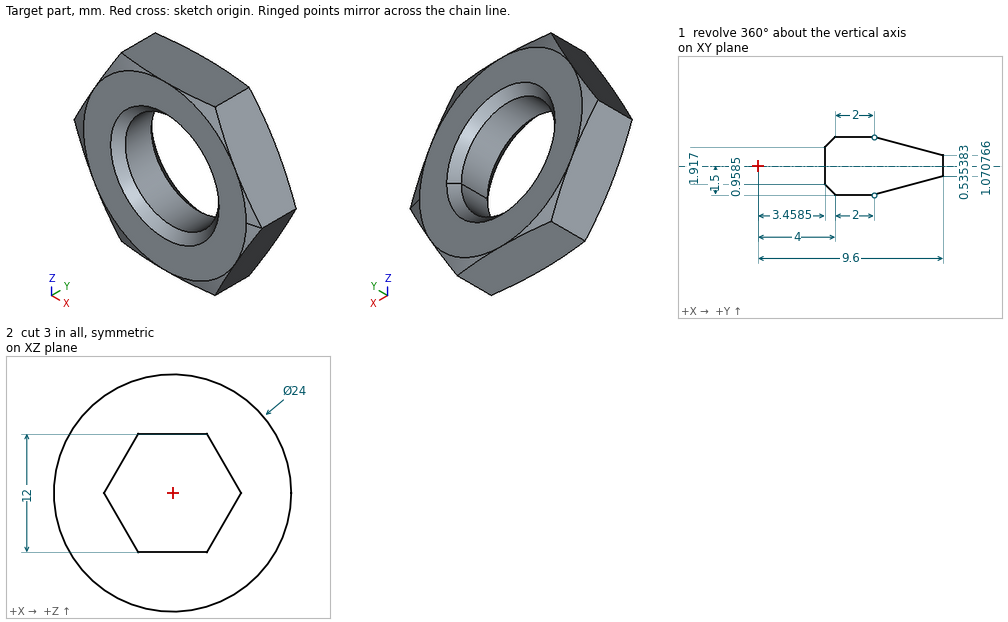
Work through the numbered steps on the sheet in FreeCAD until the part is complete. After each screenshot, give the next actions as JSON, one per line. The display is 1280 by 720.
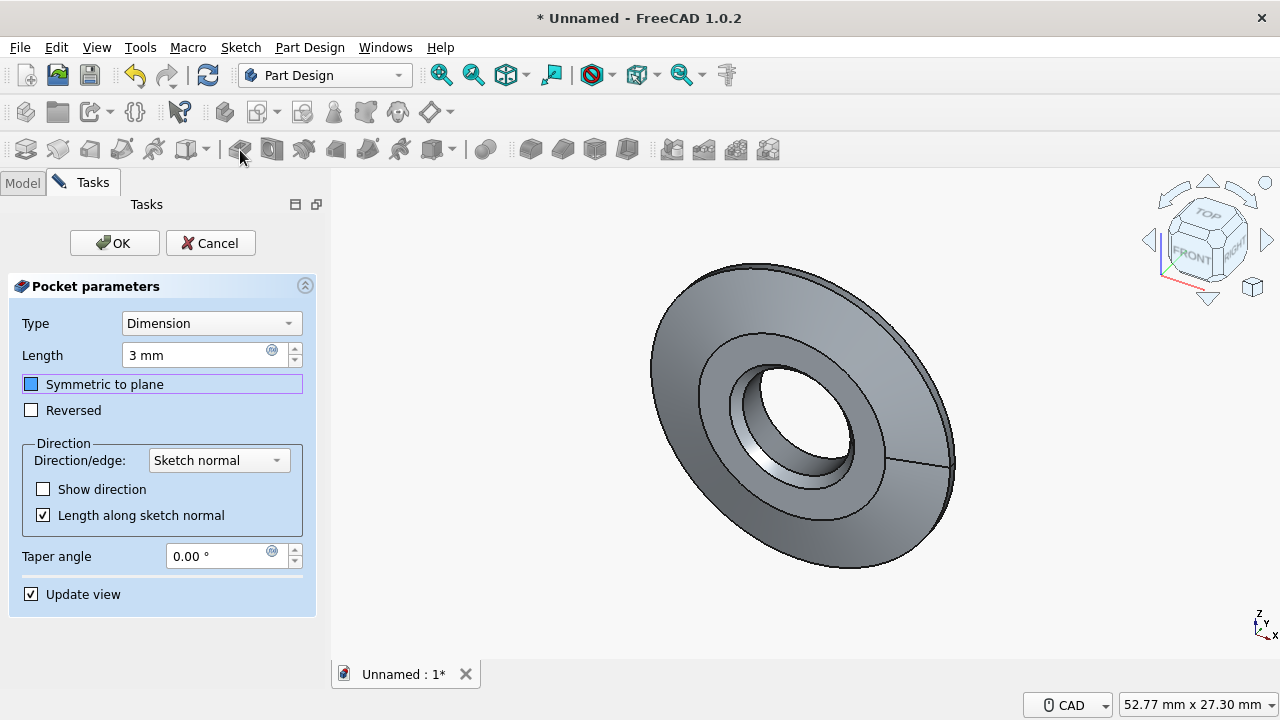
{"action": "left_click", "coordinate": [30, 384]}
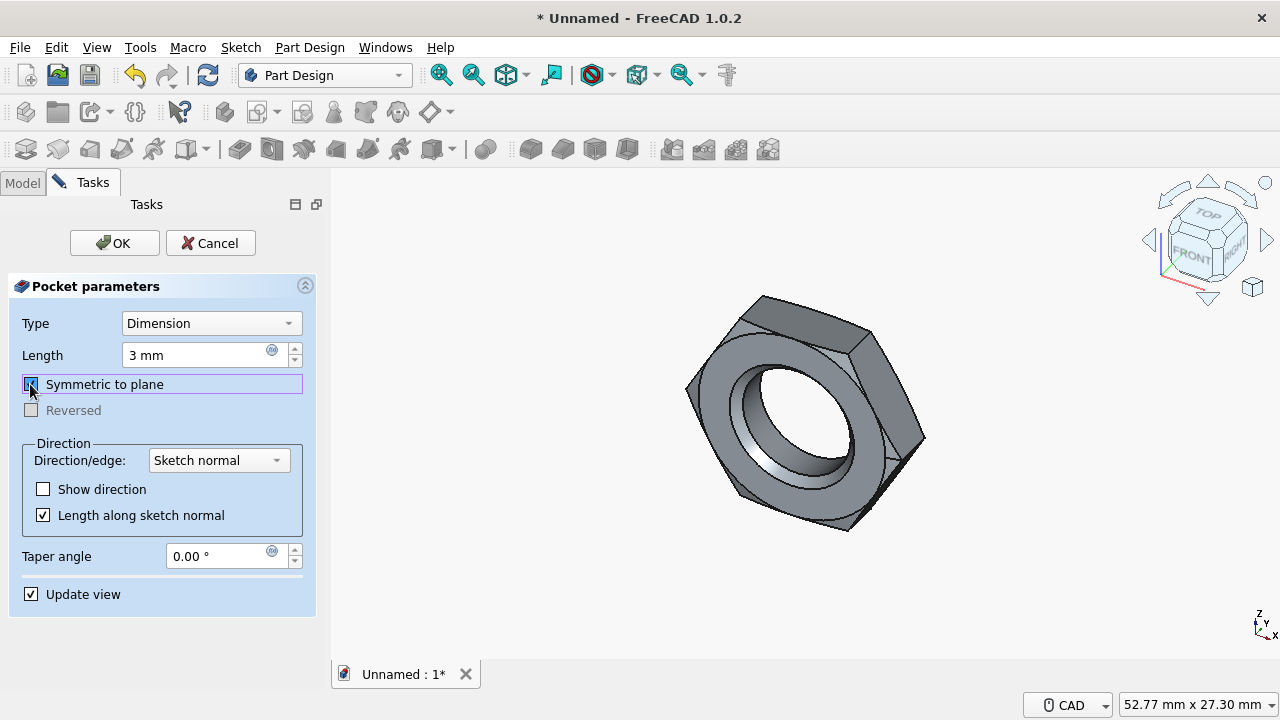
{"action": "left_click", "coordinate": [115, 243]}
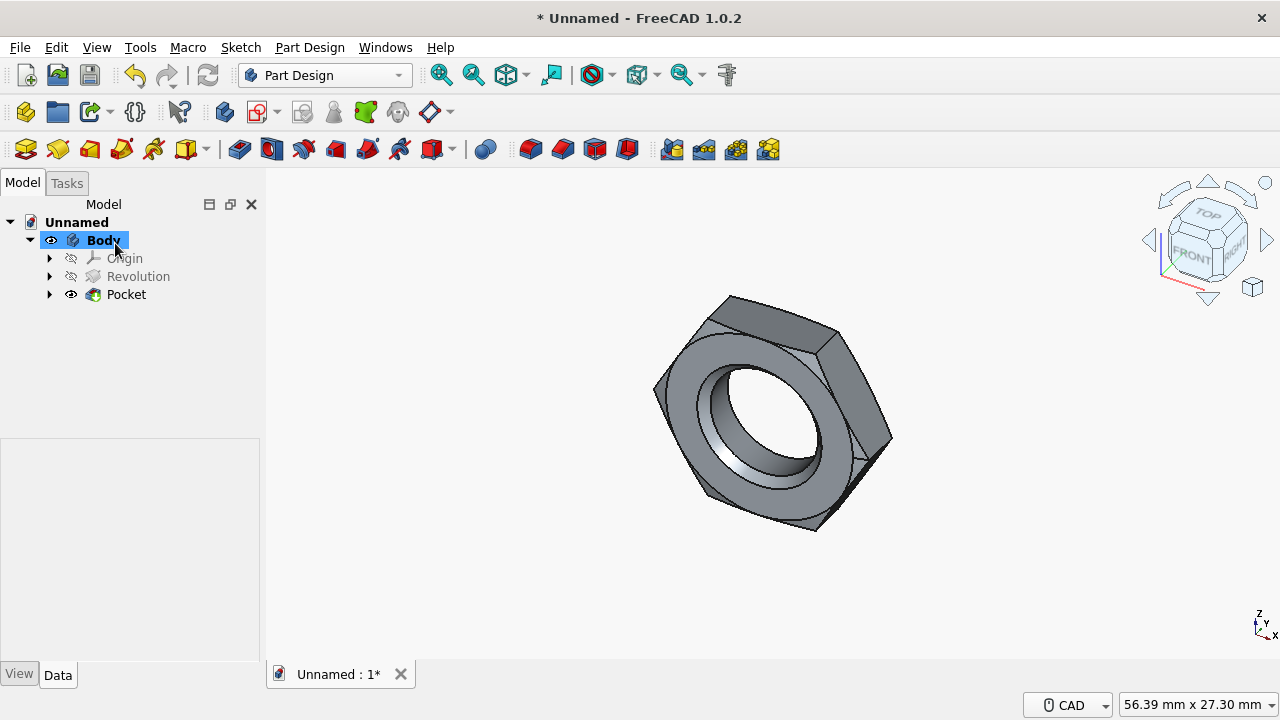
{"action": "key", "text": "0"}